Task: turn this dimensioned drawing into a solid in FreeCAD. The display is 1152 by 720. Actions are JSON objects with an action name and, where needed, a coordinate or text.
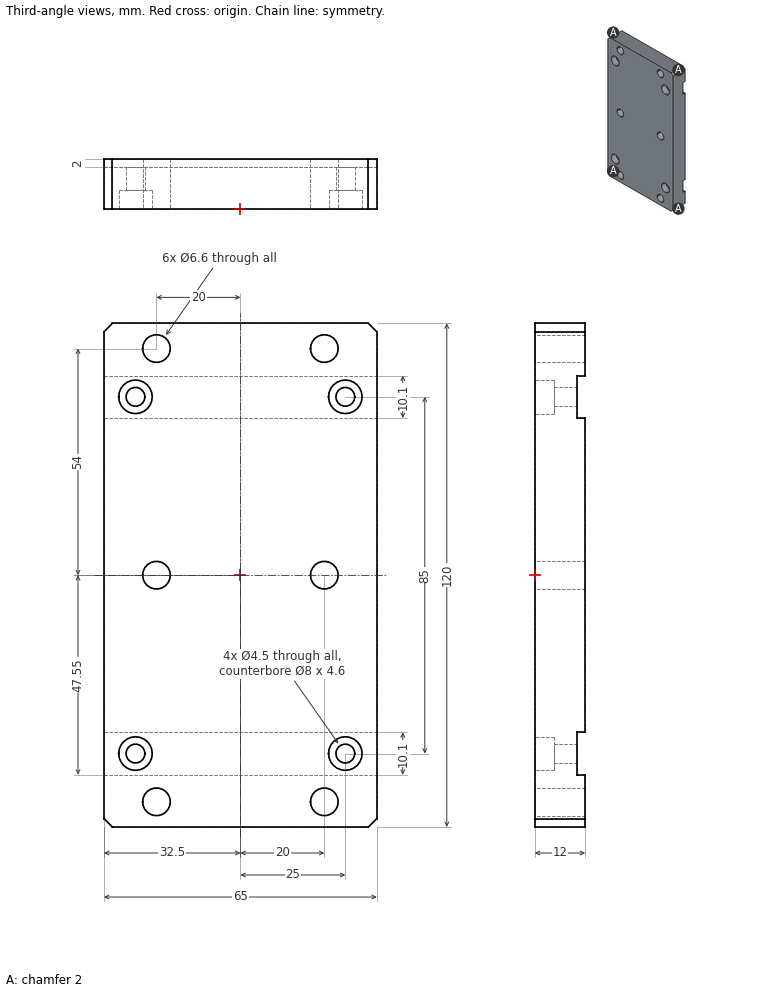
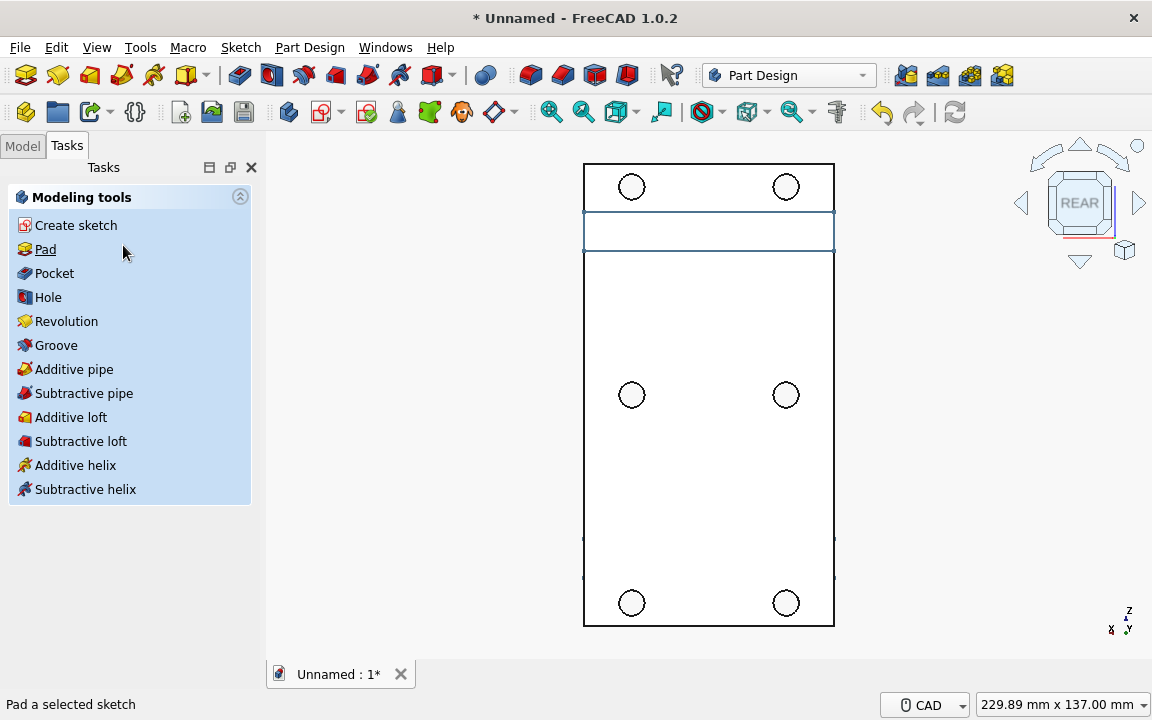
{"action": "left_click", "coordinate": [240, 76]}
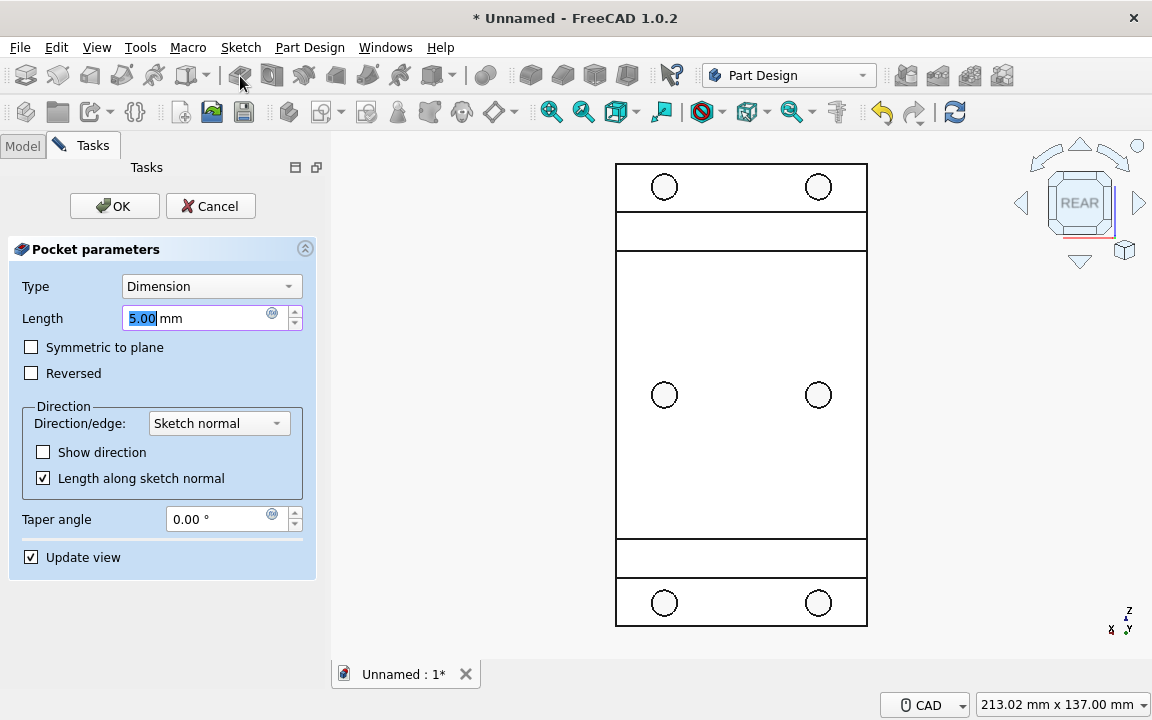
{"action": "type", "text": "2"}
{"action": "key", "text": "Tab"}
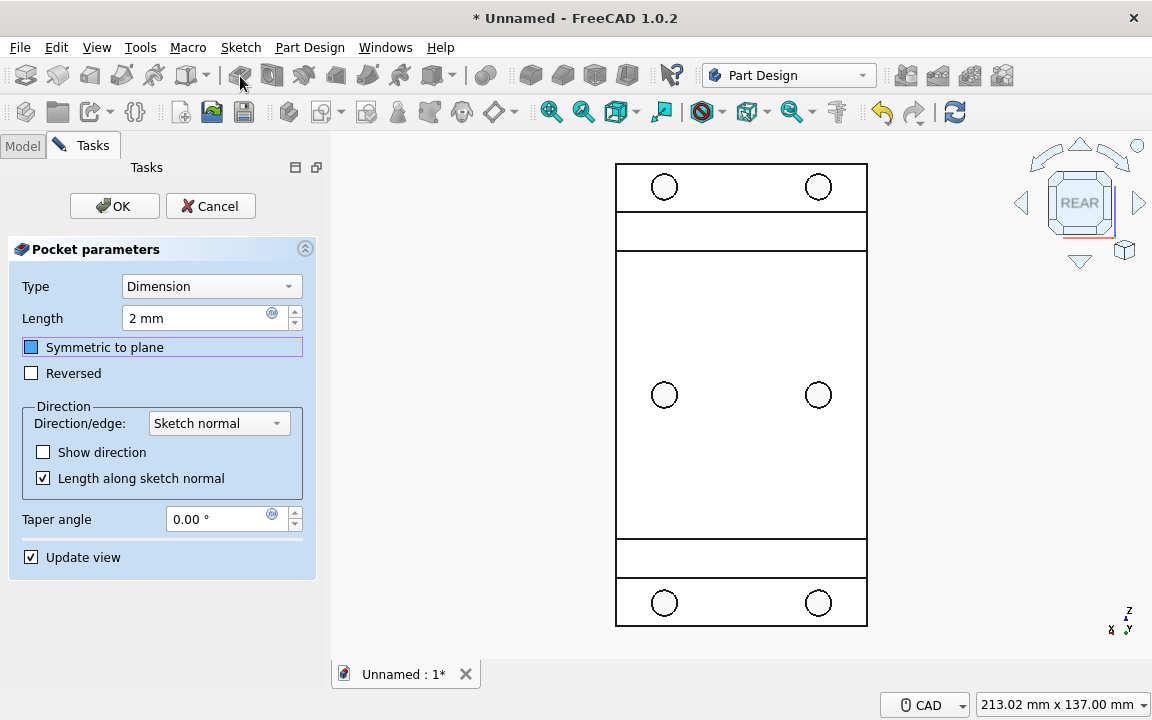
{"action": "left_click", "coordinate": [115, 206]}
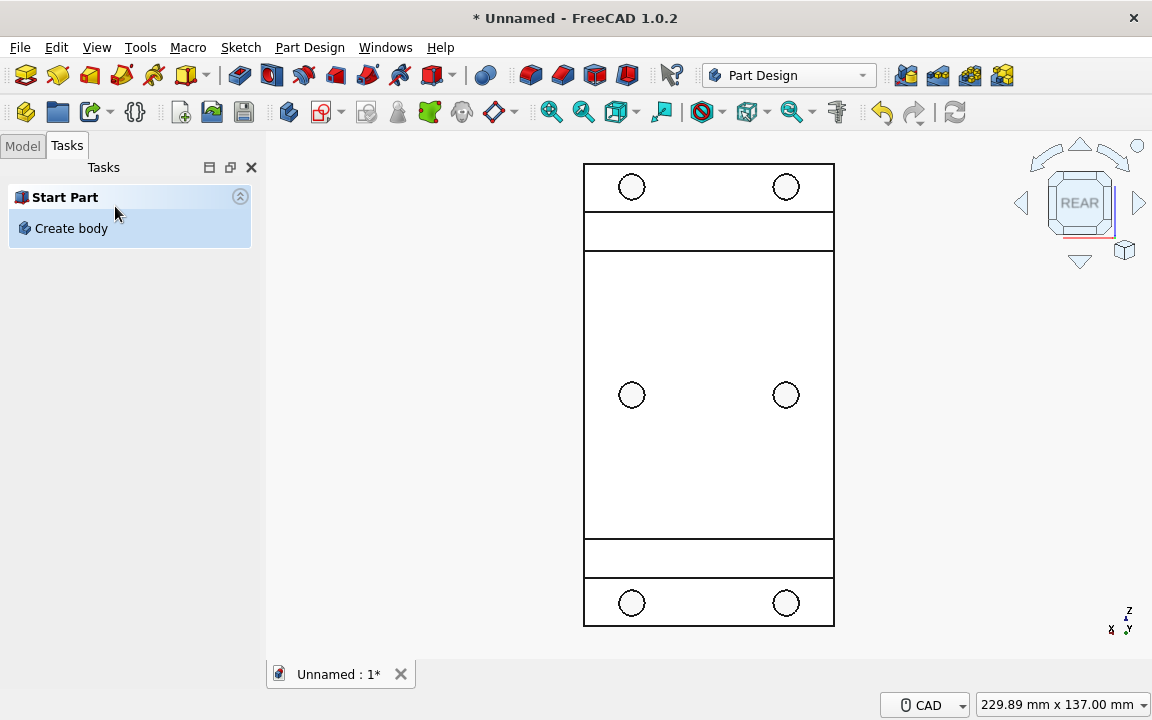
{"action": "key", "text": "0"}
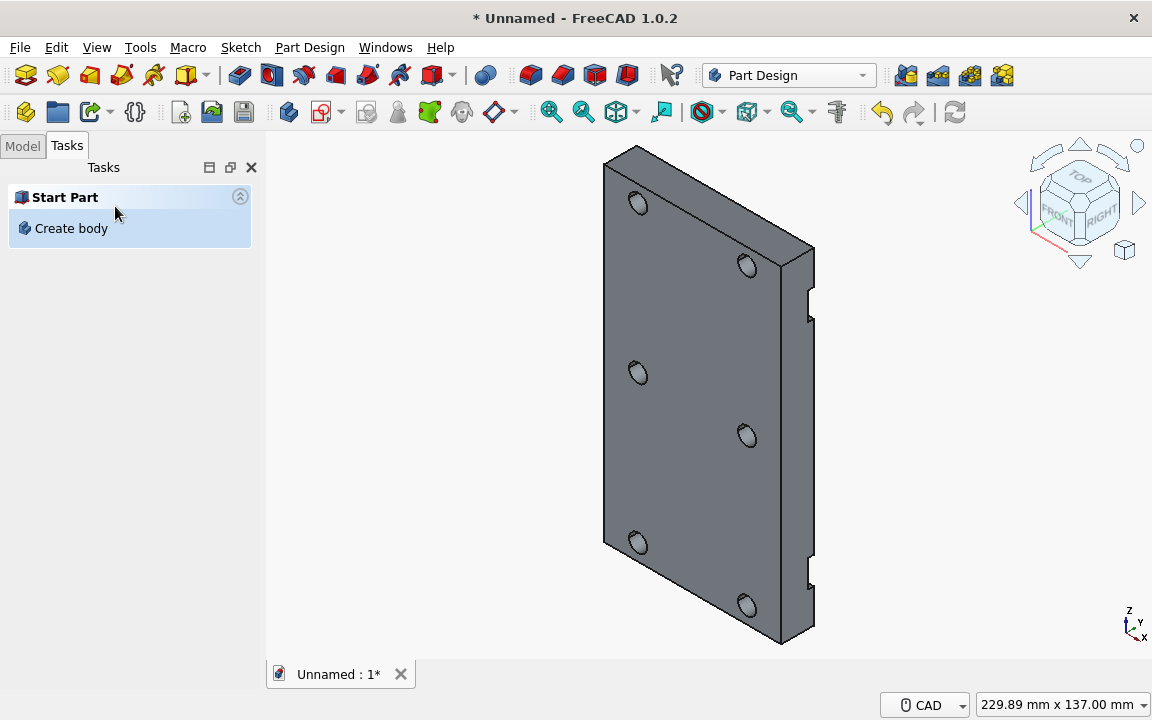
{"action": "left_click", "coordinate": [798, 256]}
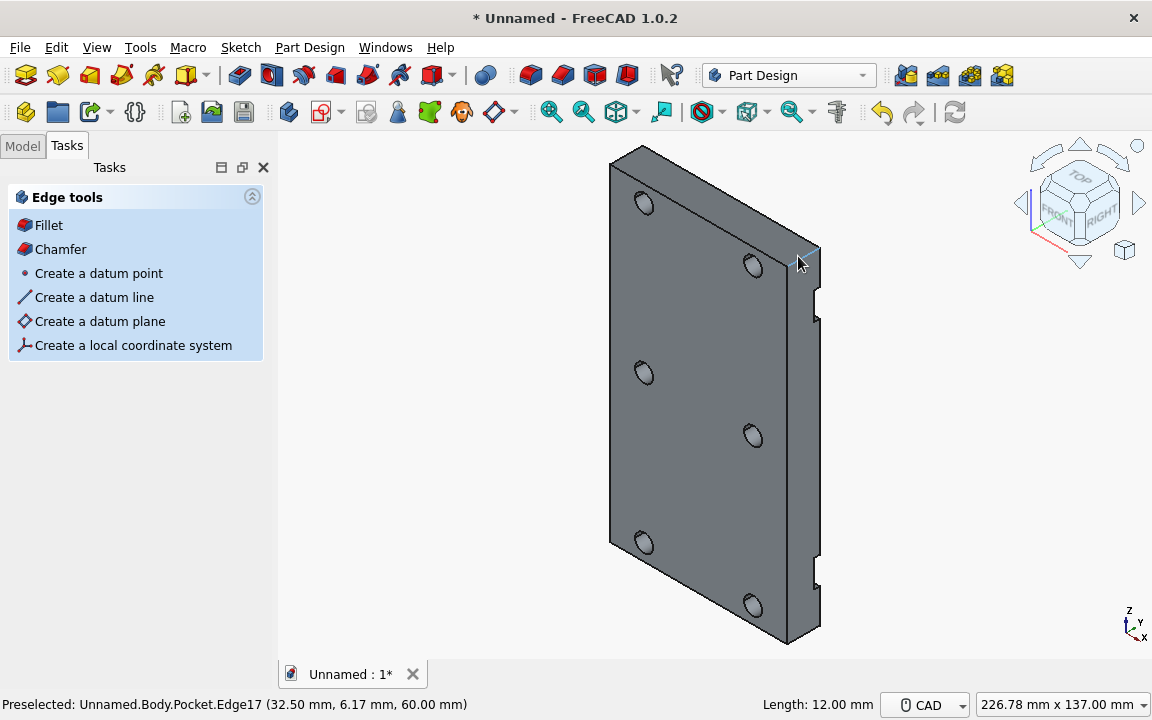
{"action": "key", "text": "2"}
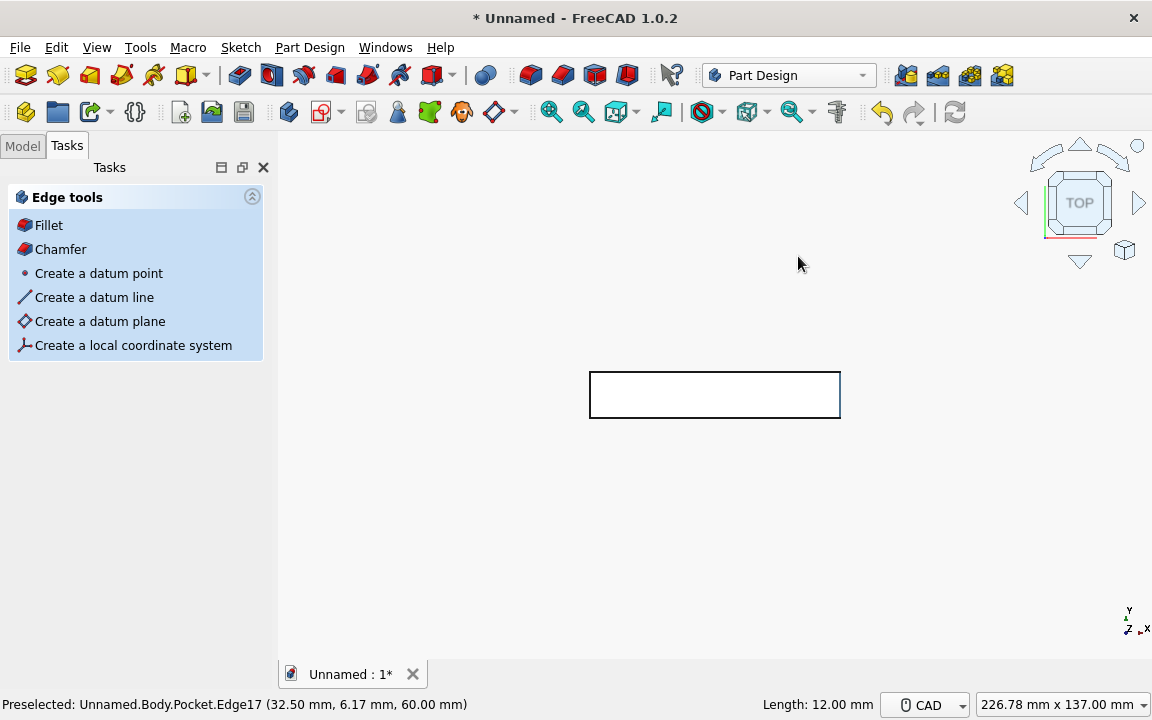
{"action": "key", "text": "v f"}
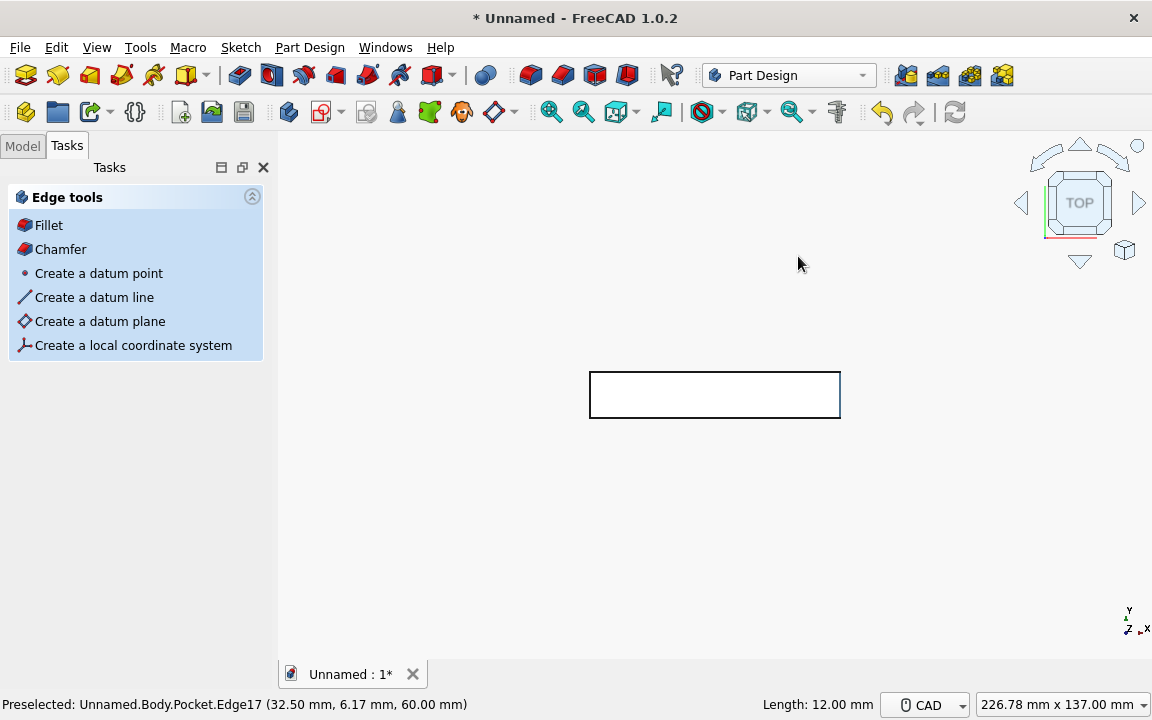
{"action": "left_click", "coordinate": [590, 394], "text": "ctrl"}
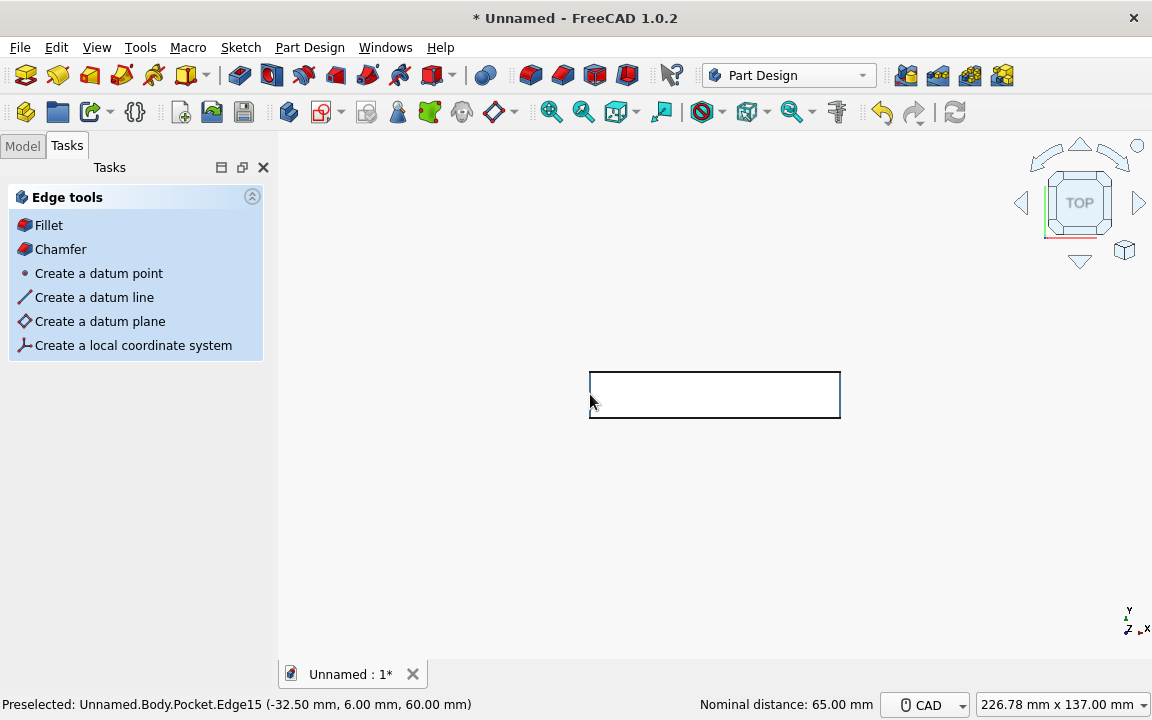
{"action": "key", "text": "1"}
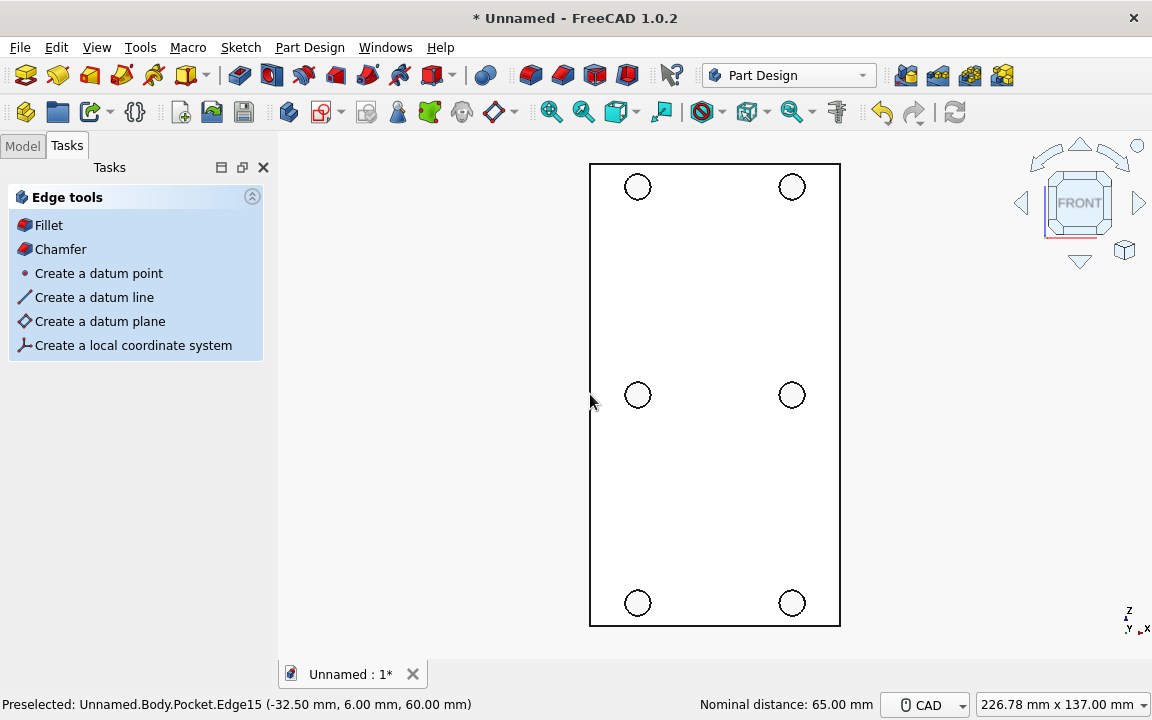
{"action": "key", "text": "3"}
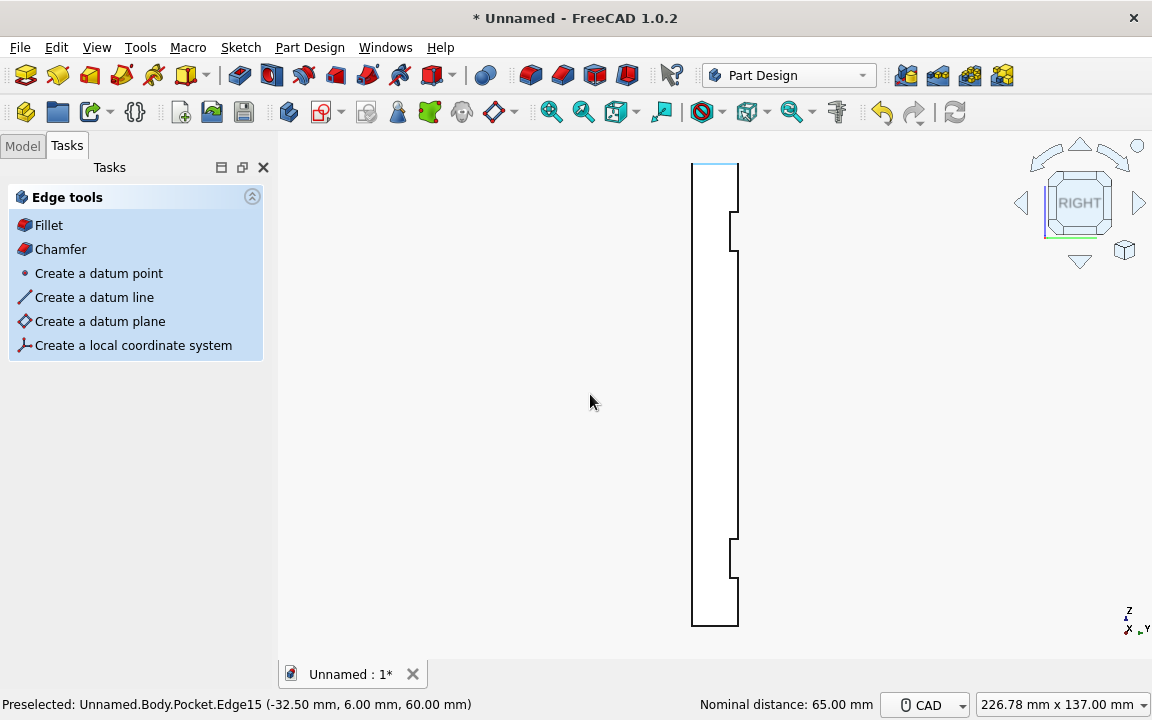
{"action": "left_click", "coordinate": [715, 625], "text": "ctrl"}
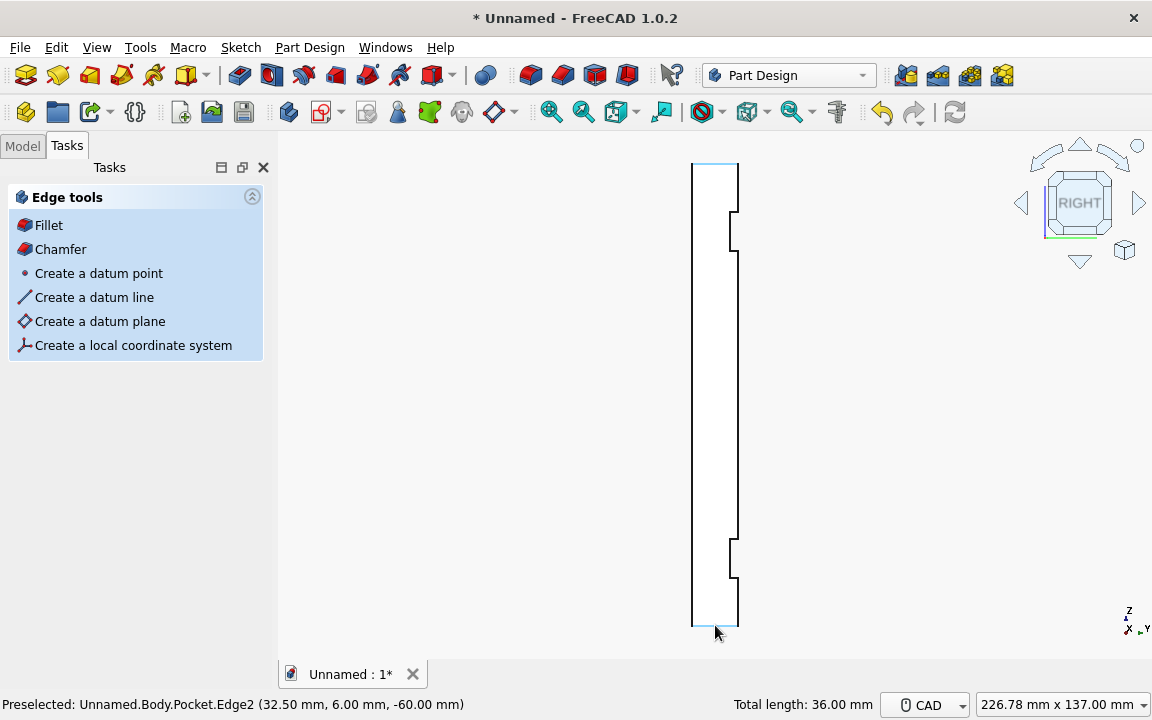
{"action": "key", "text": "5"}